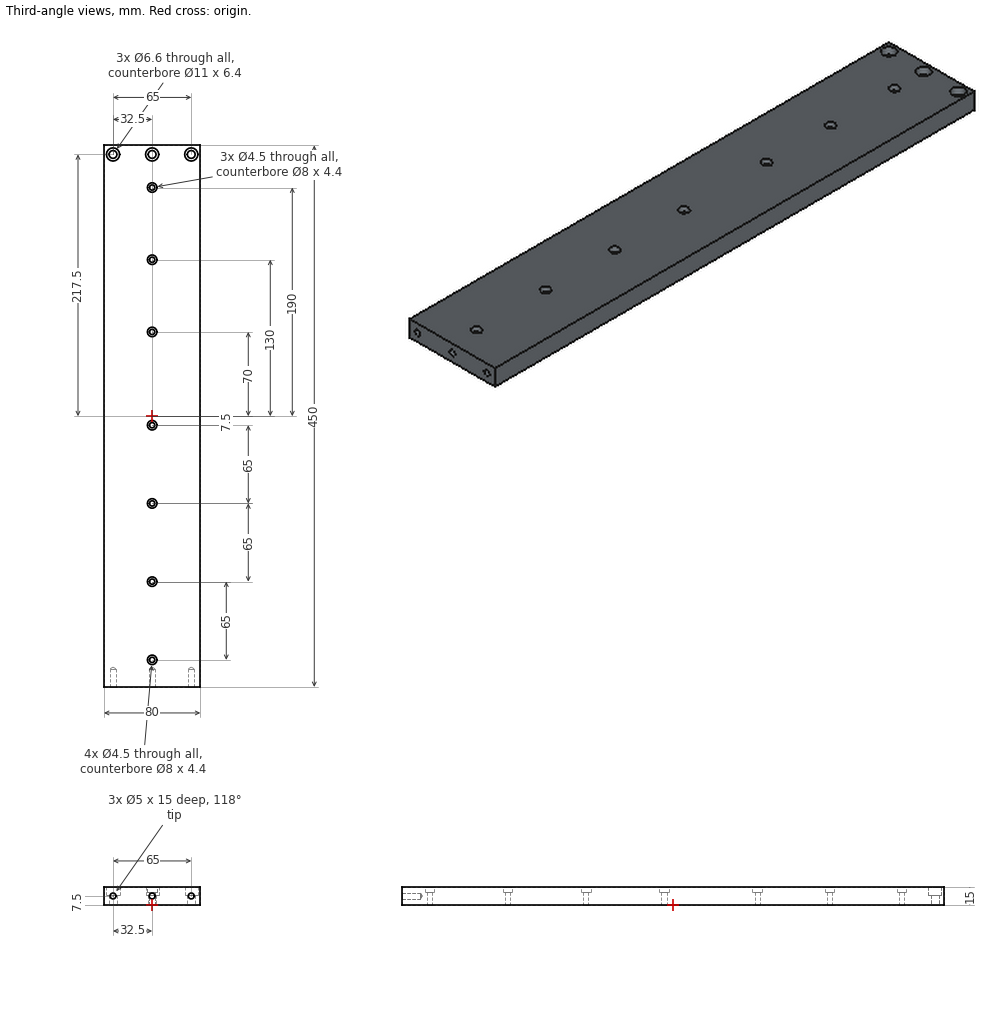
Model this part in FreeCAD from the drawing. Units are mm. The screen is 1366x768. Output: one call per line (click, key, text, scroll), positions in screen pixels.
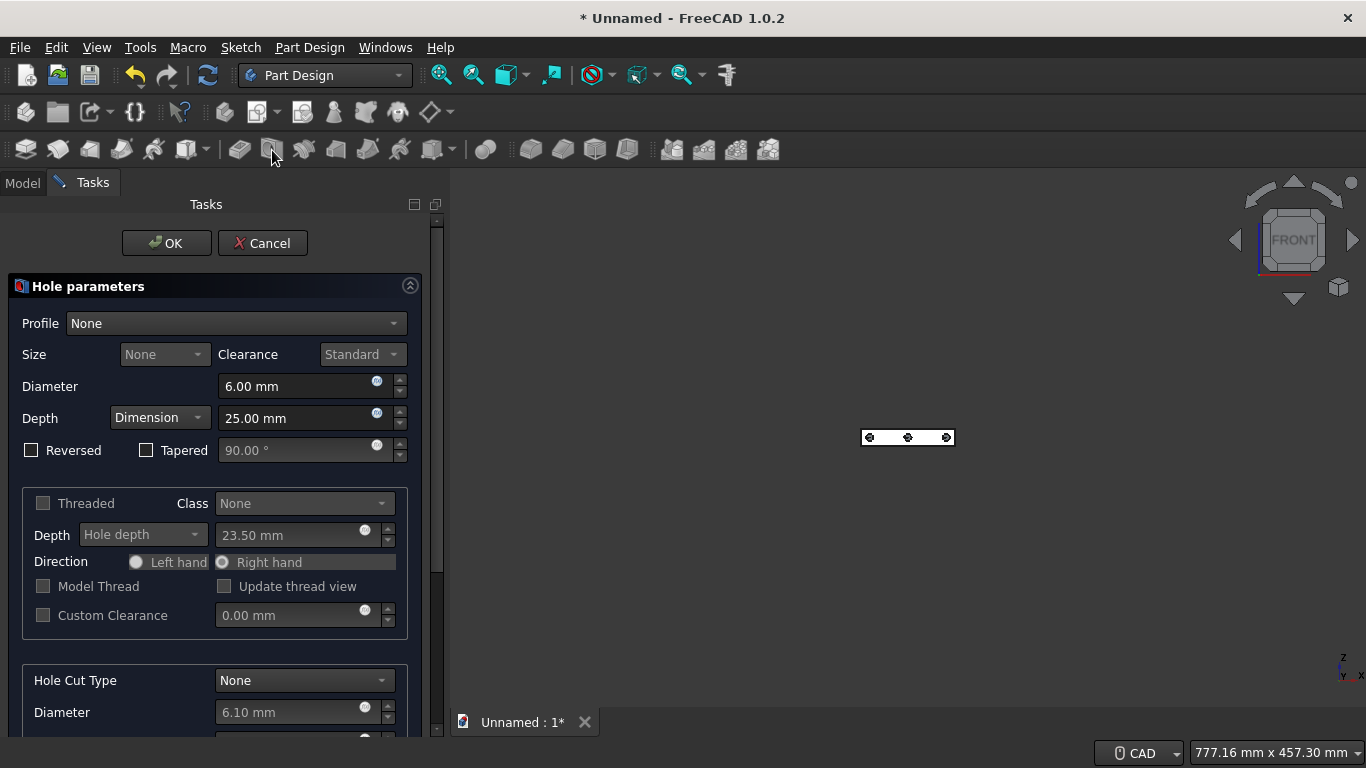
triple_click(305, 386)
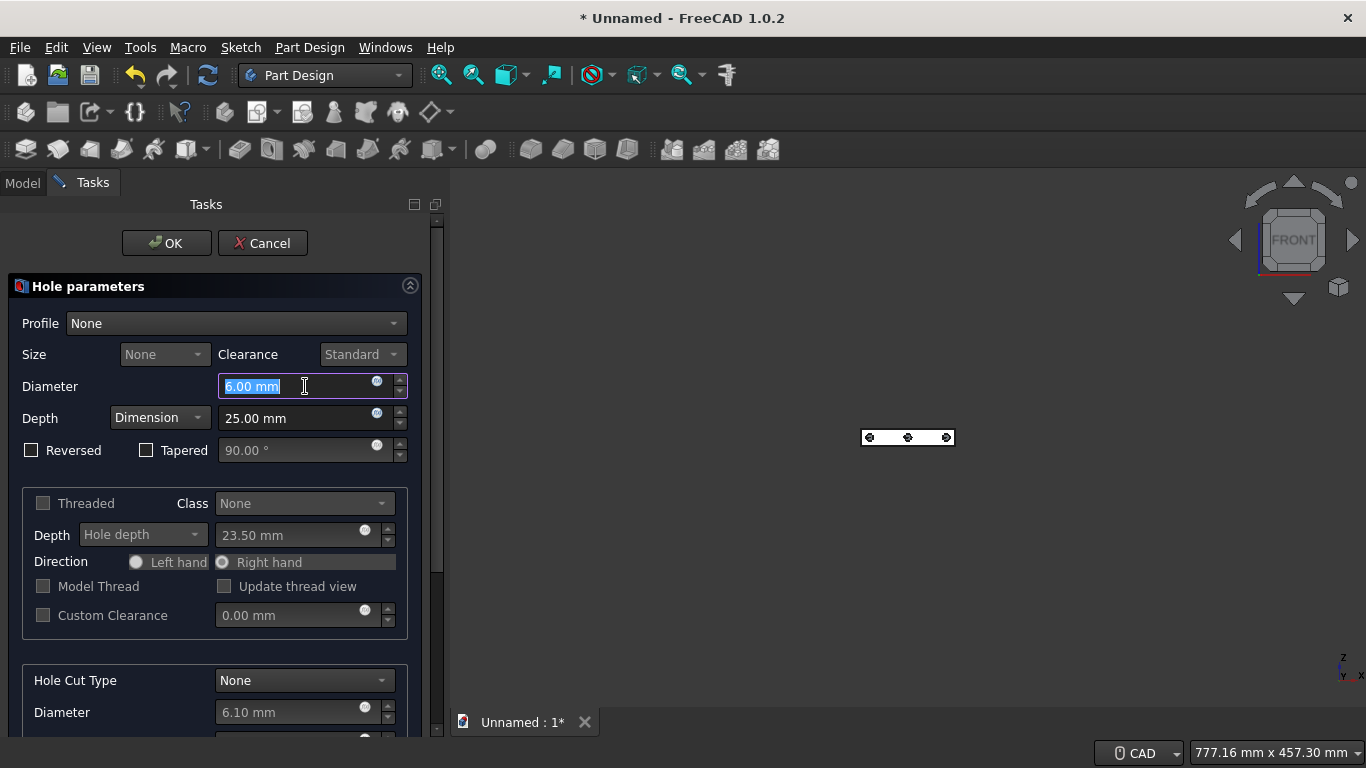
text(5)
key(Tab)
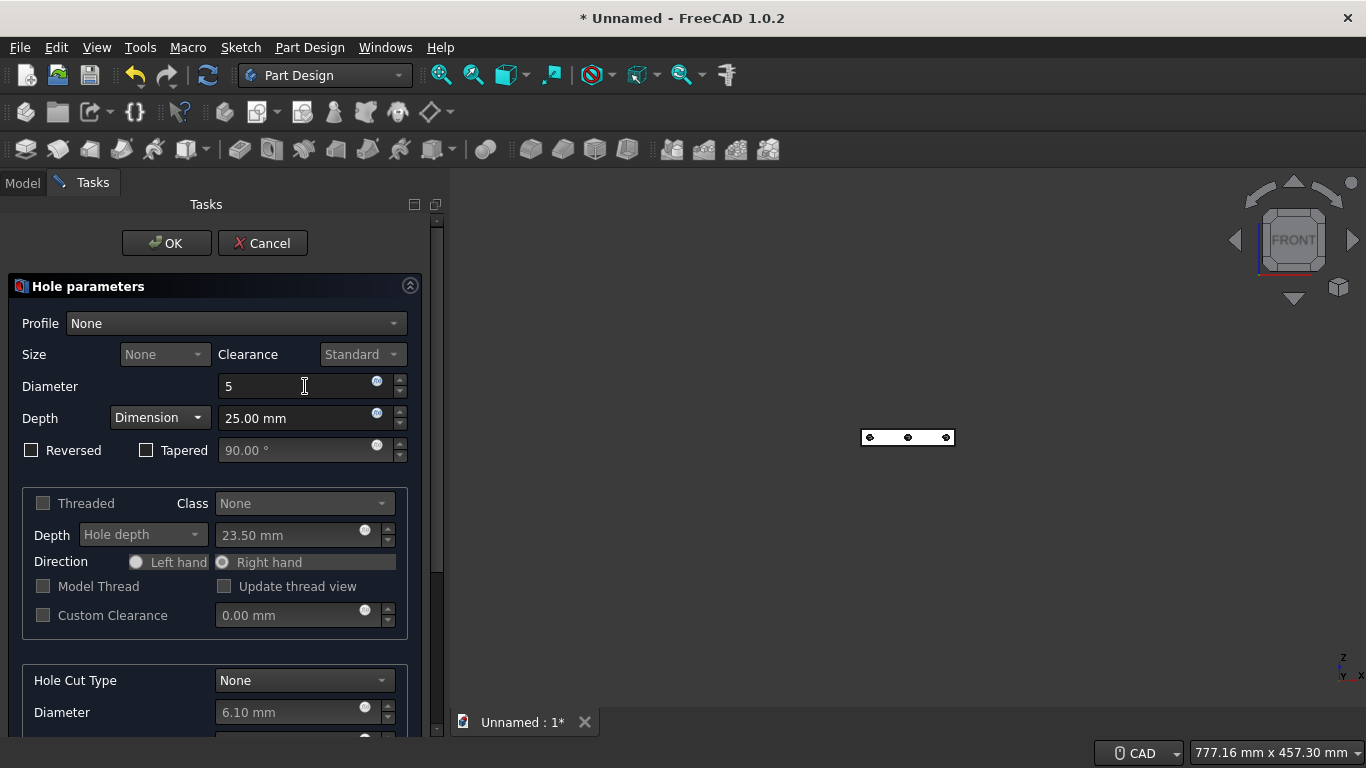
triple_click(305, 418)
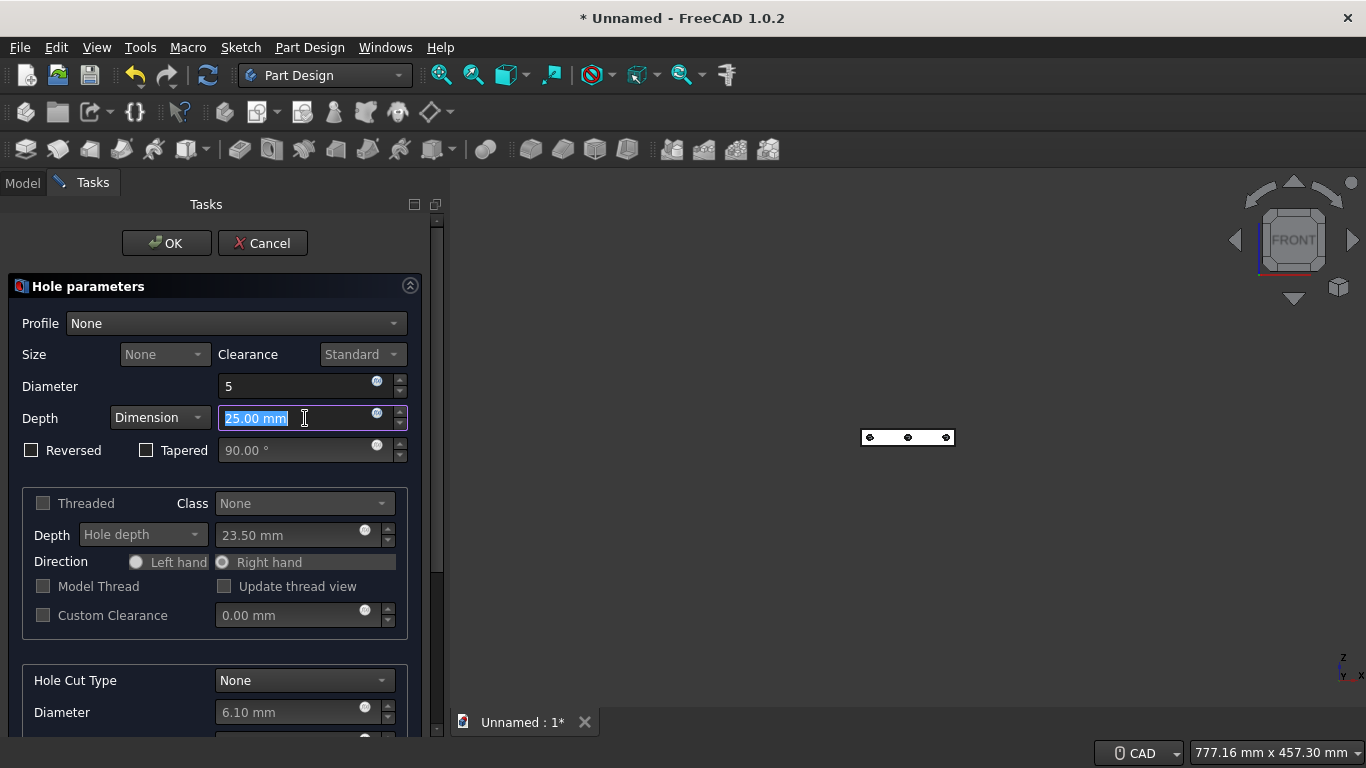
text(15)
key(Tab)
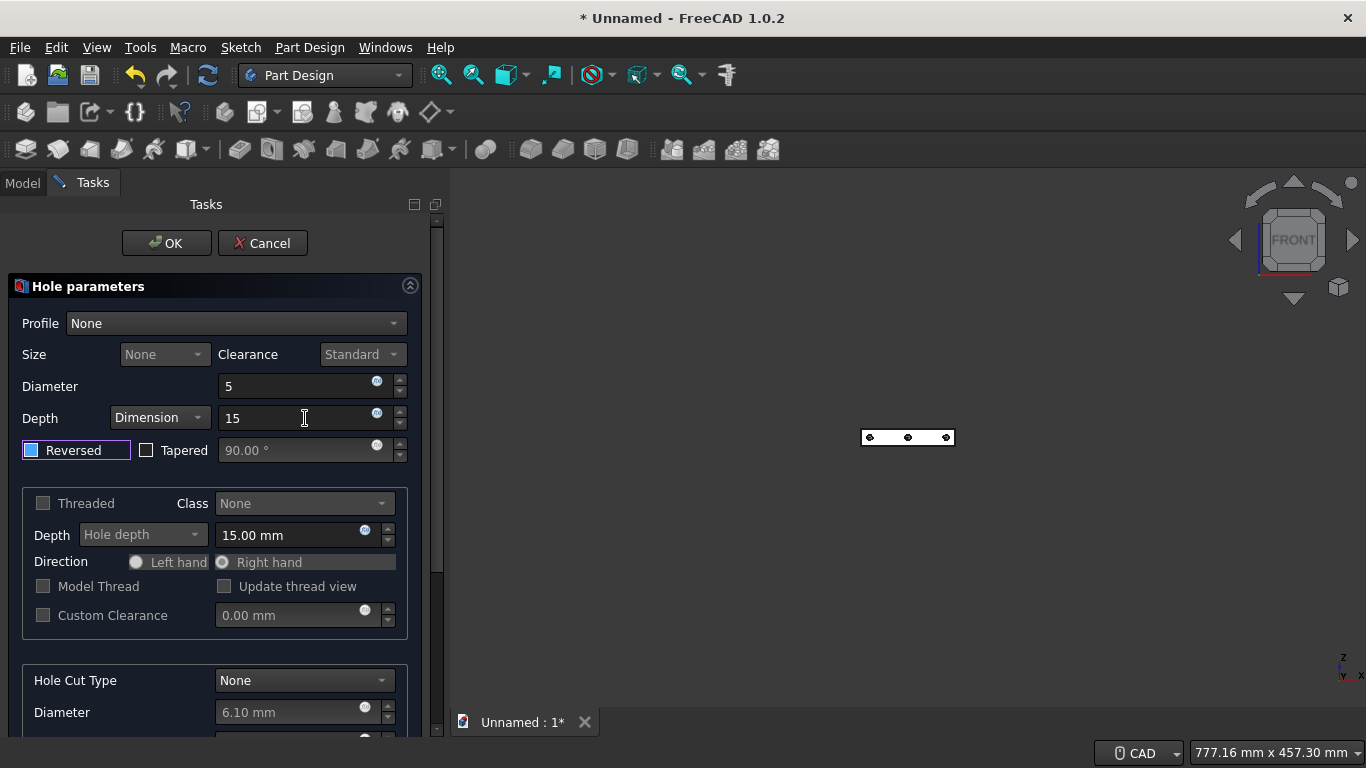
click(167, 243)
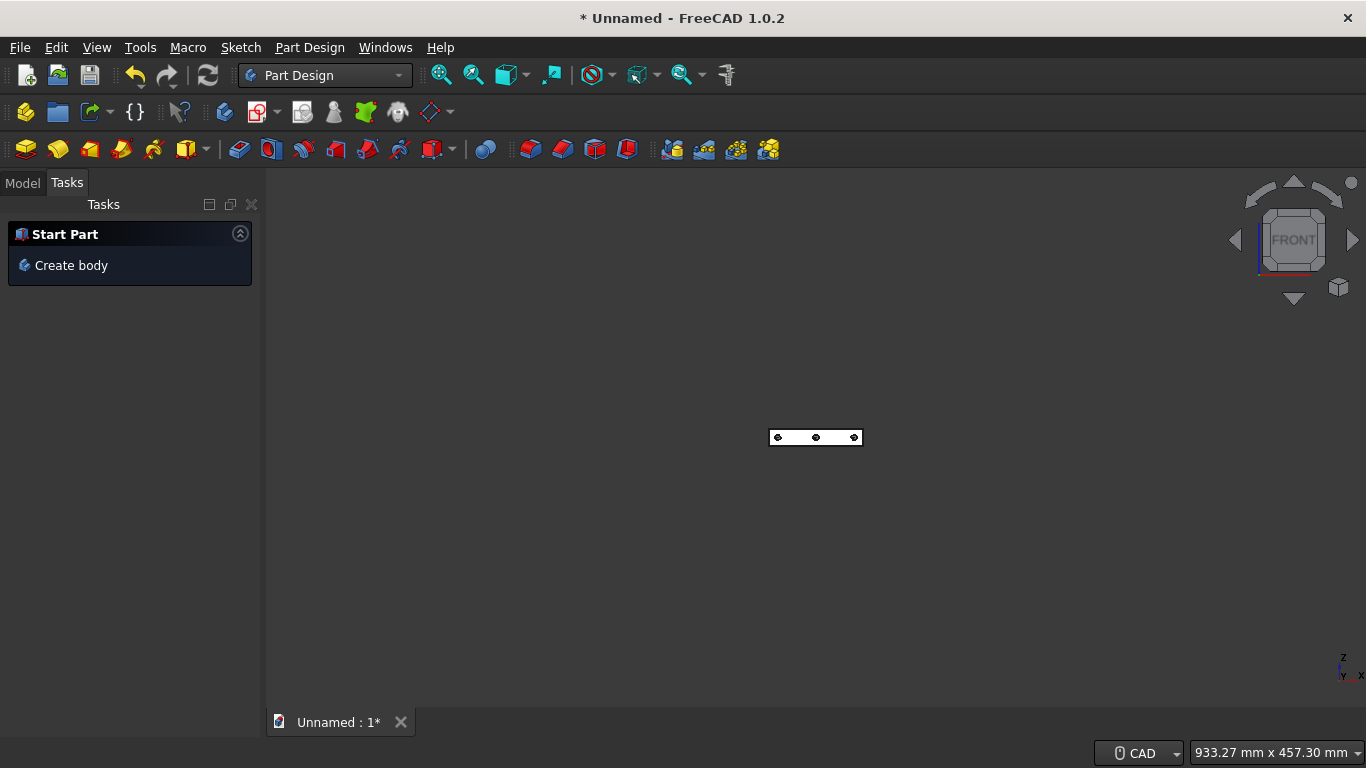
key(0)